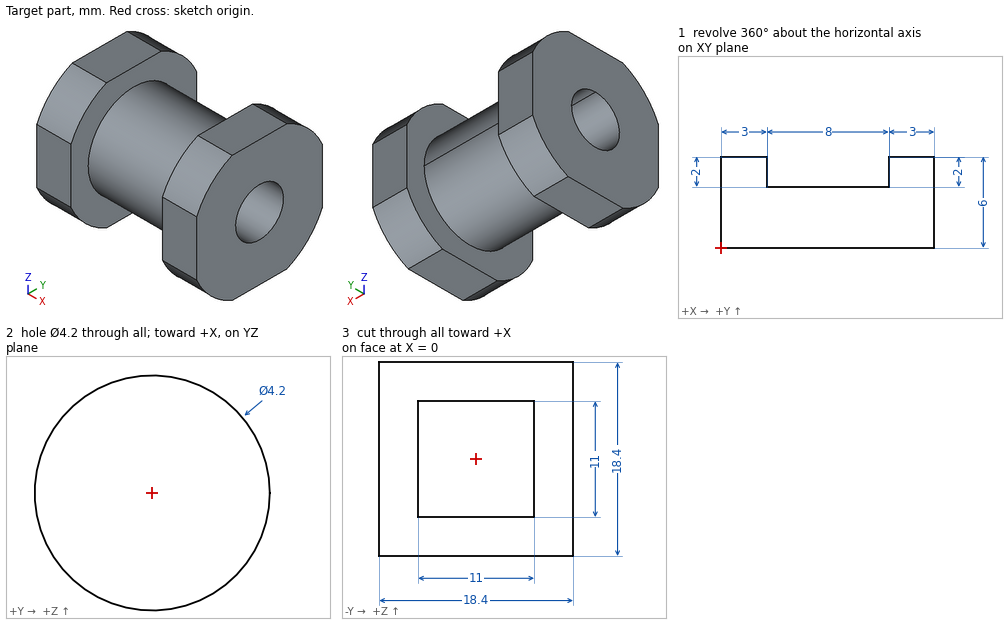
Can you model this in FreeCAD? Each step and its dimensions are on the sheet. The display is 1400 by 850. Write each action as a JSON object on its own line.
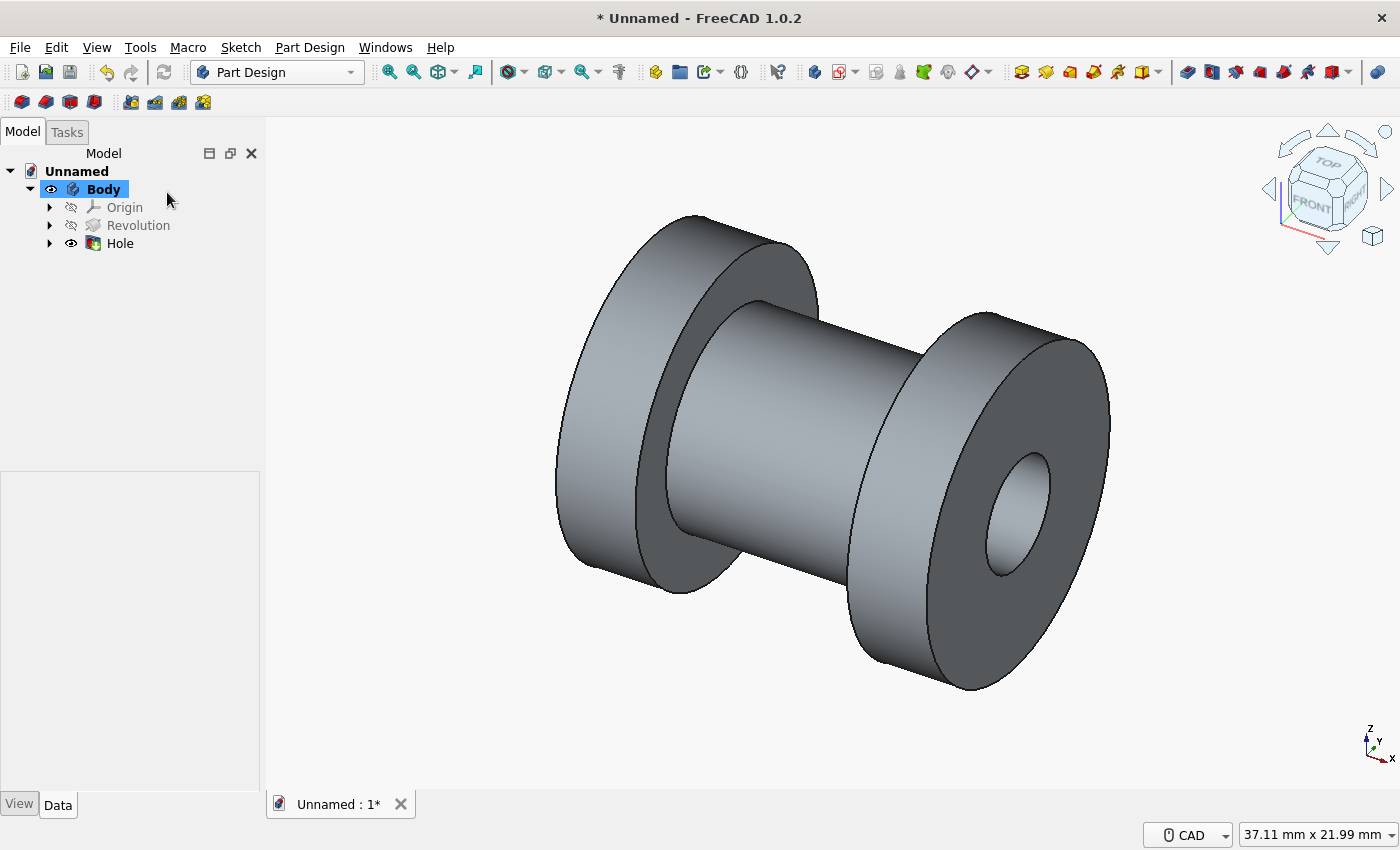
{"action": "key", "text": "6"}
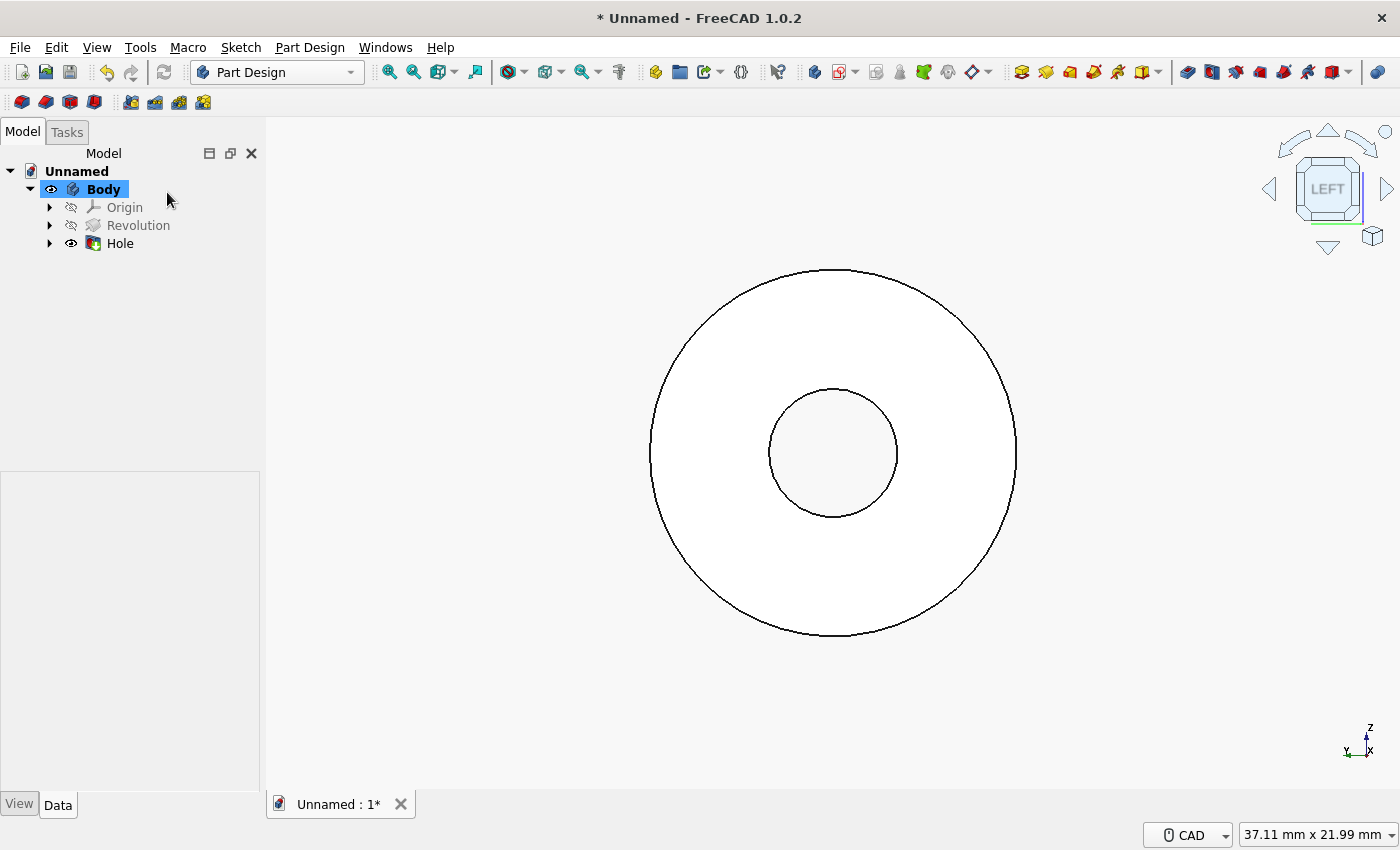
{"action": "left_click", "coordinate": [728, 504]}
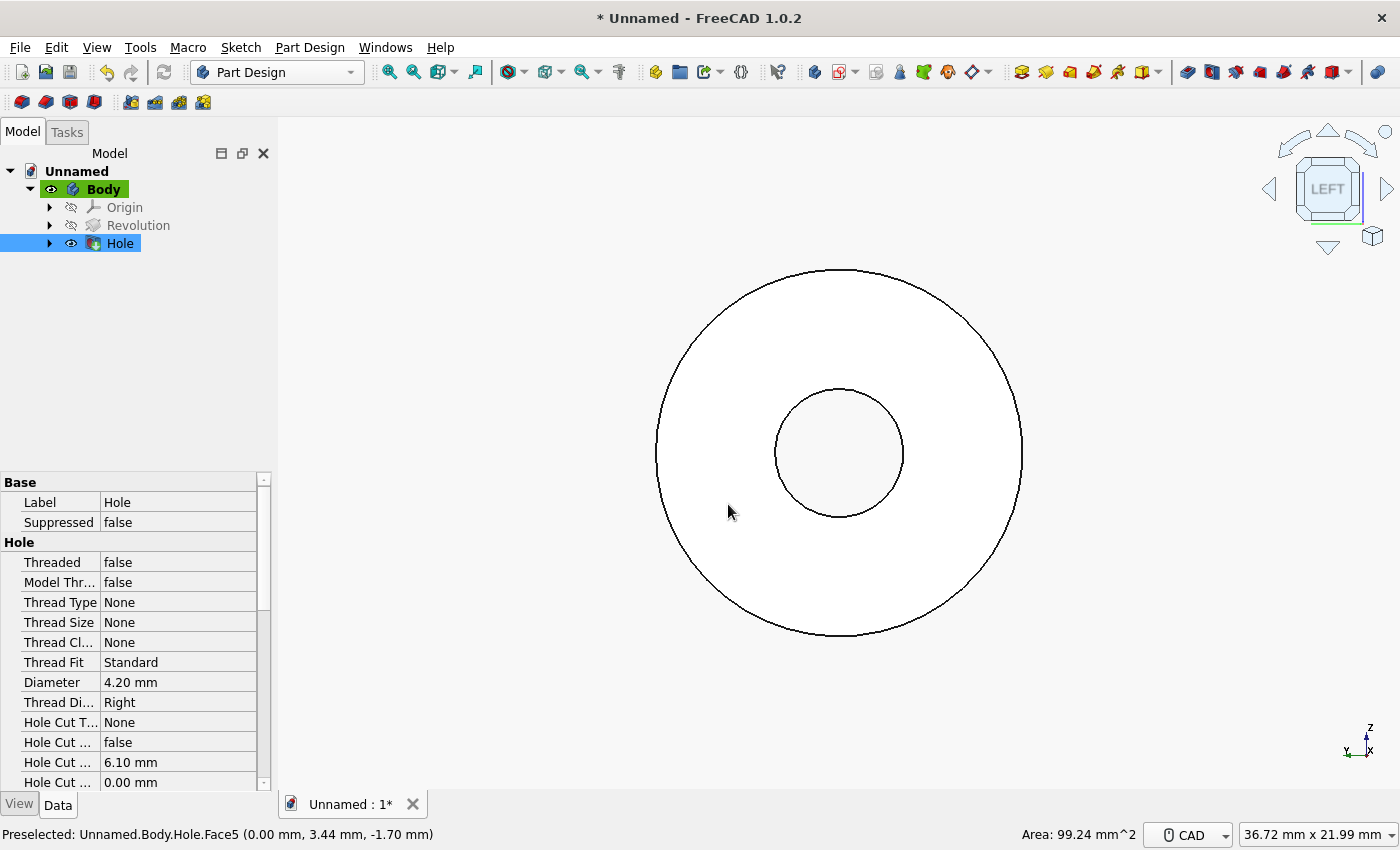
{"action": "left_click", "coordinate": [840, 72]}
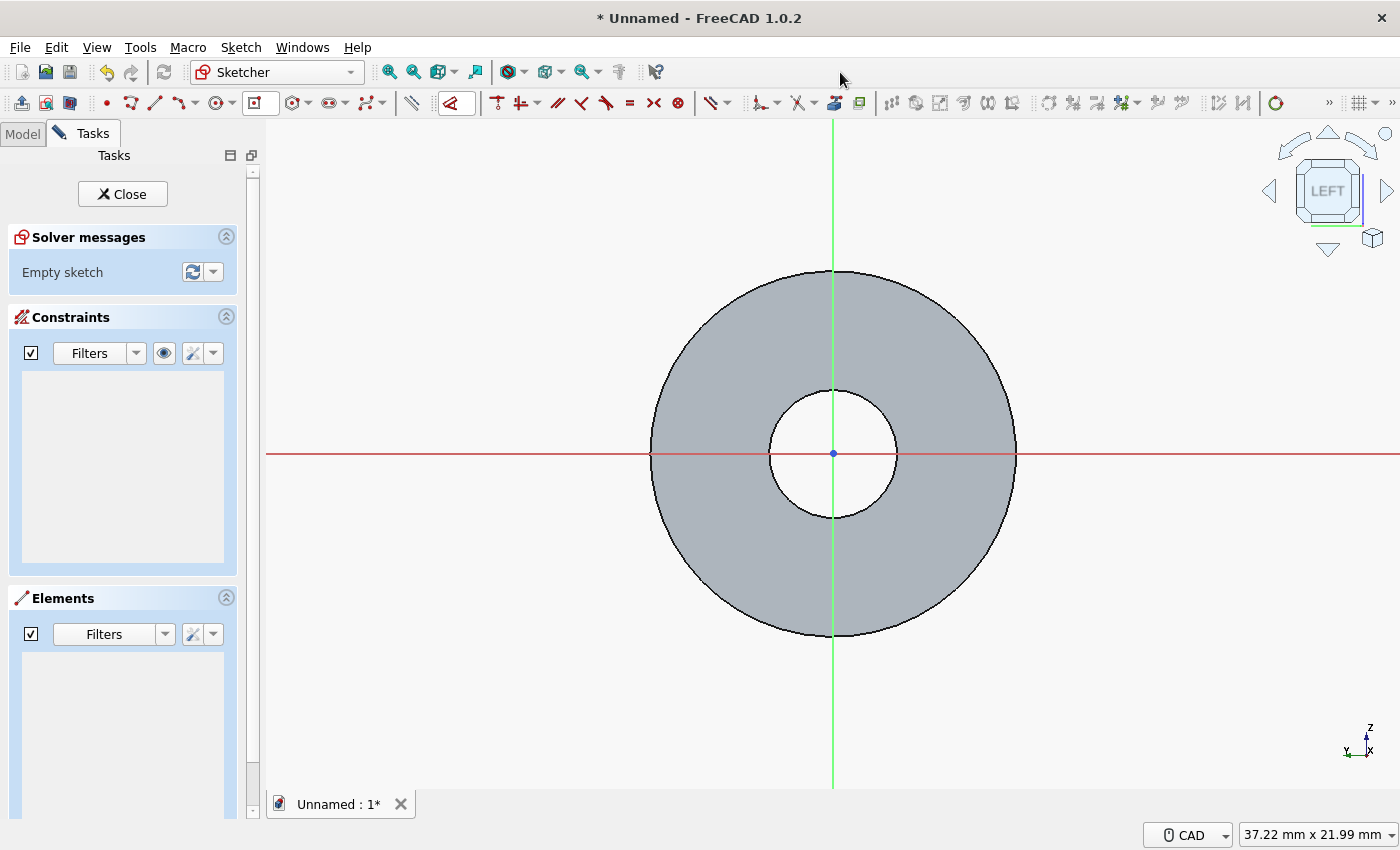
{"action": "left_click", "coordinate": [254, 104]}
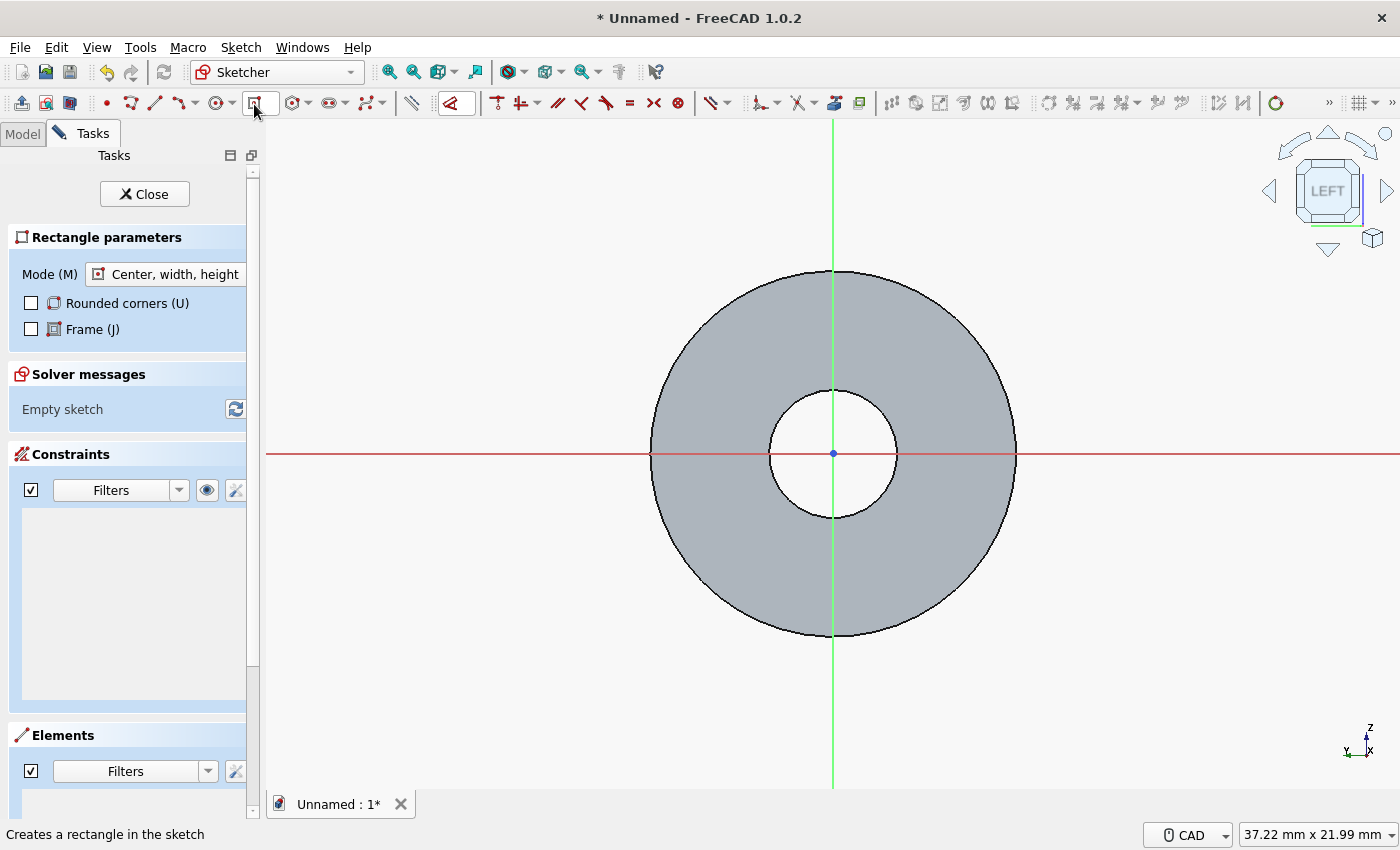
{"action": "left_click", "coordinate": [833, 454]}
{"action": "mouse_move", "coordinate": [1113, 174]}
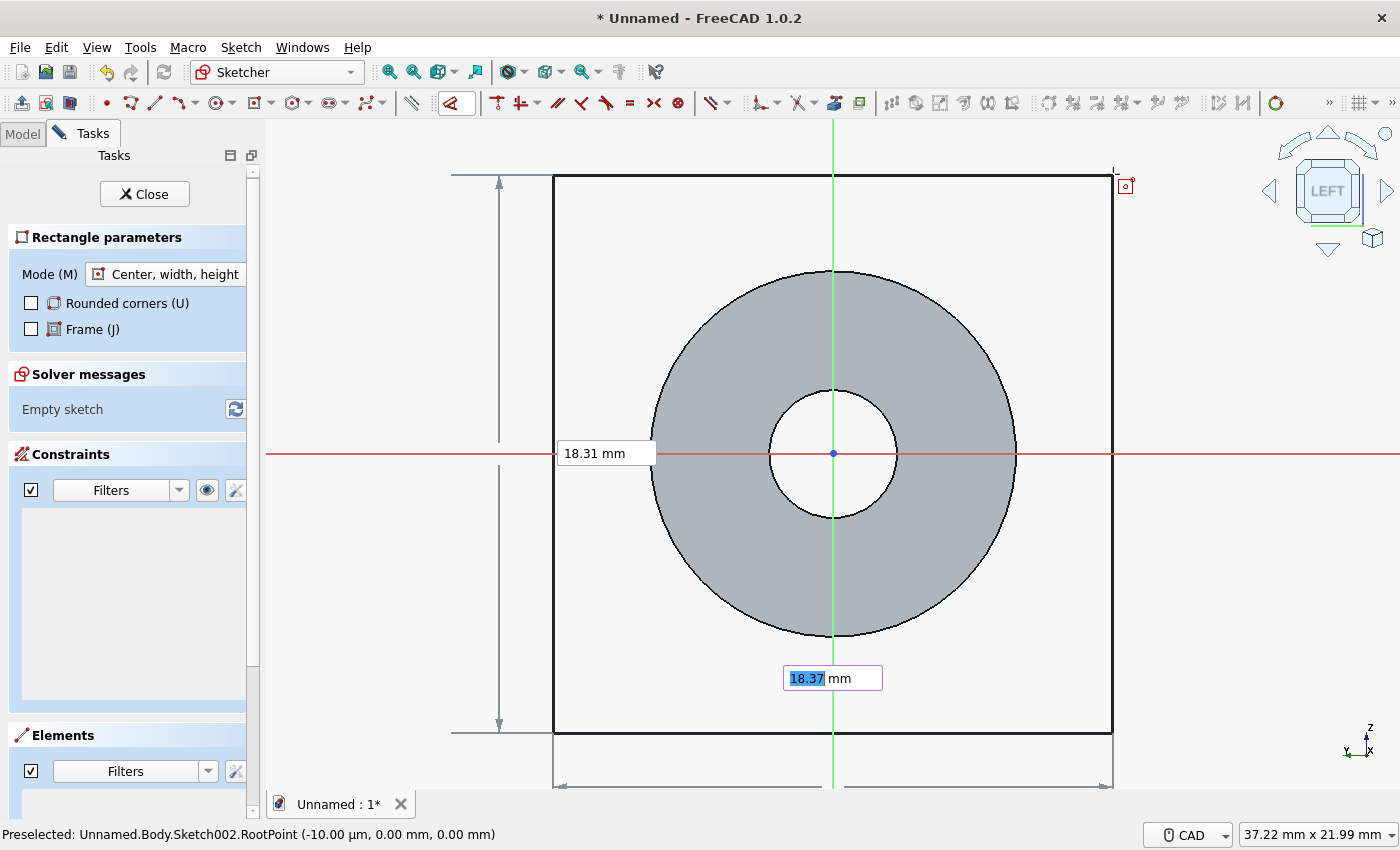
{"action": "type", "text": "18.4"}
{"action": "key", "text": "Tab"}
{"action": "type", "text": "18.4"}
{"action": "key", "text": "Return"}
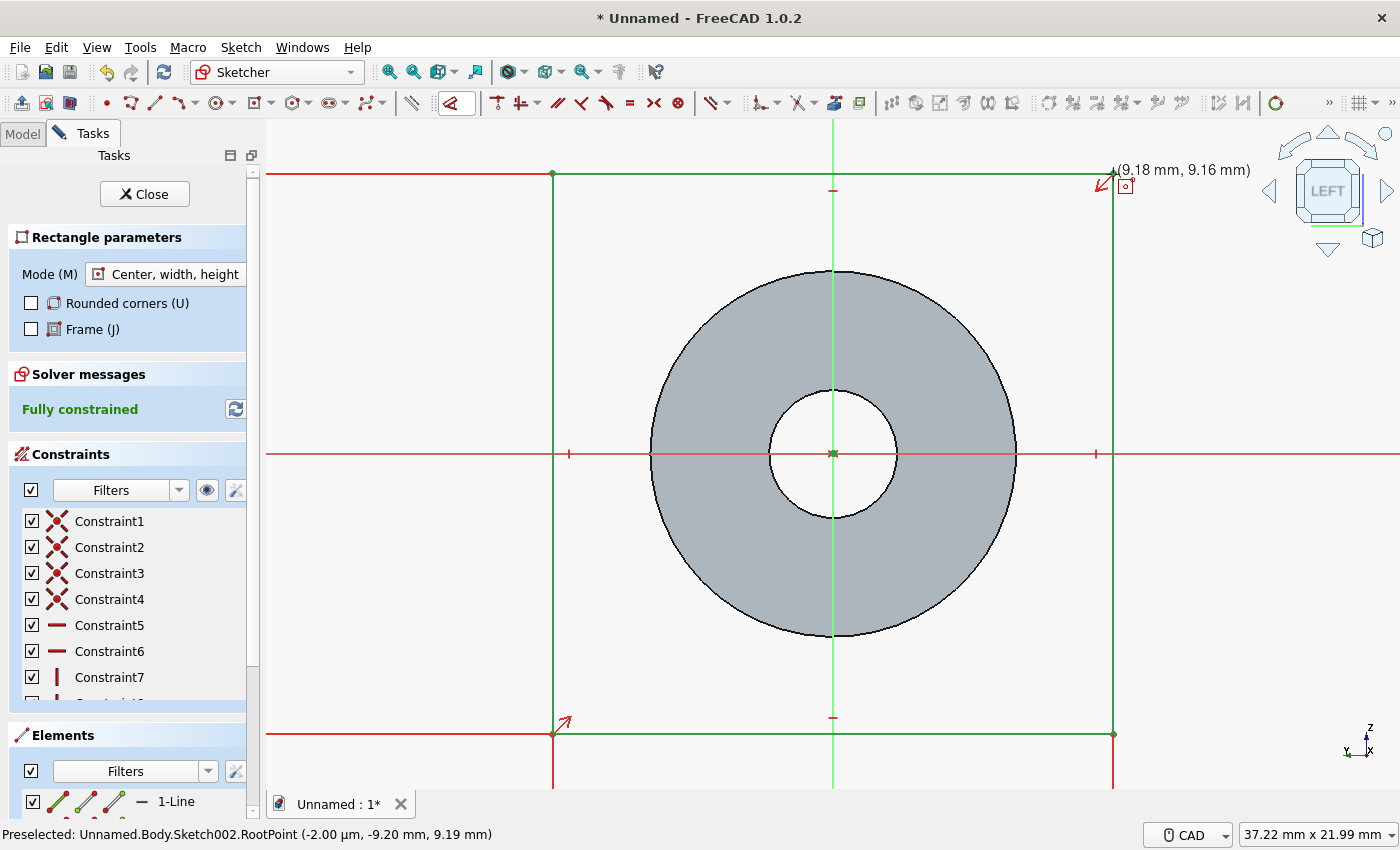
{"action": "left_click", "coordinate": [833, 454]}
{"action": "mouse_move", "coordinate": [1001, 286]}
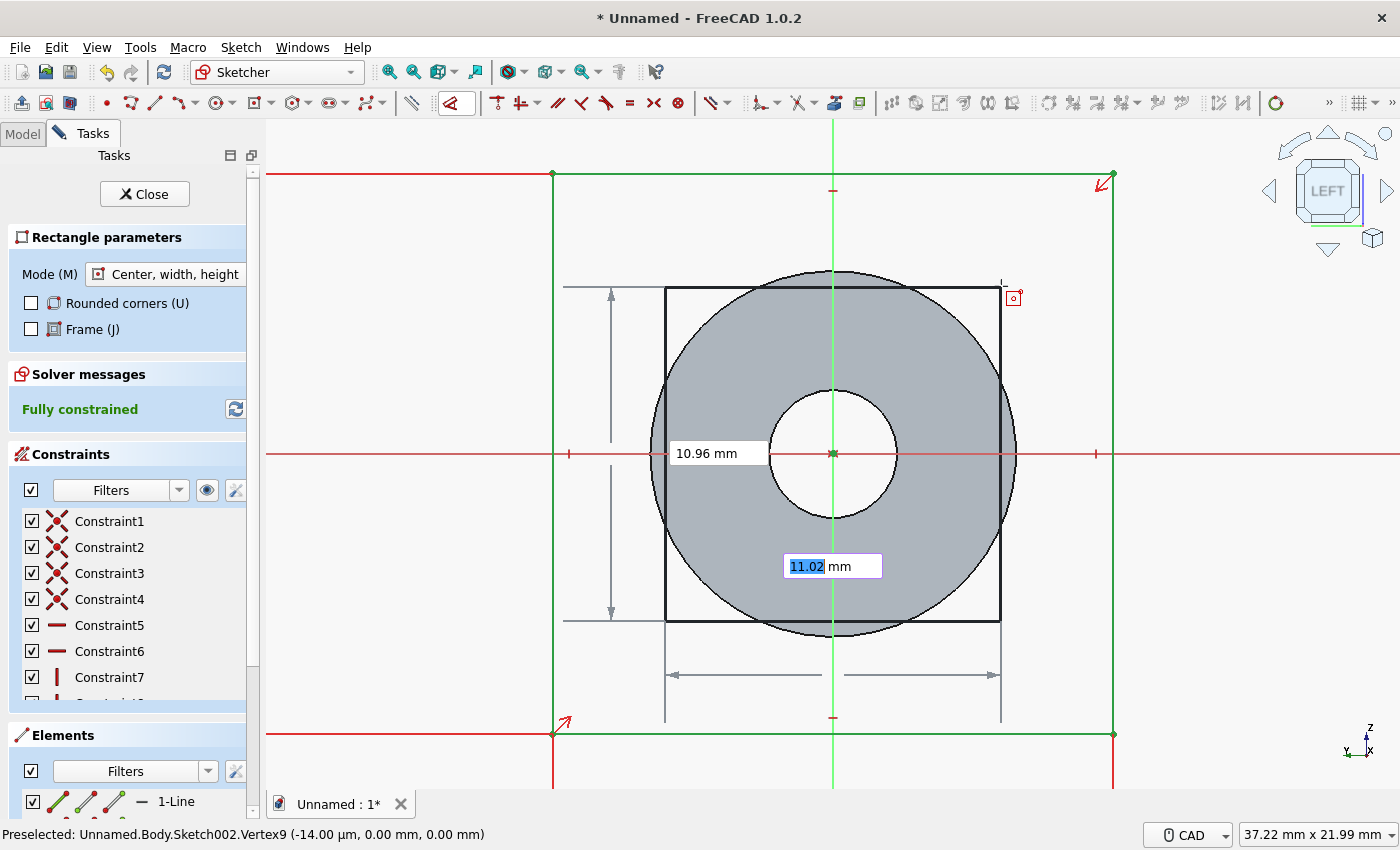
{"action": "type", "text": "11"}
{"action": "key", "text": "Tab"}
{"action": "type", "text": "11"}
{"action": "key", "text": "Return"}
{"action": "key", "text": "Escape"}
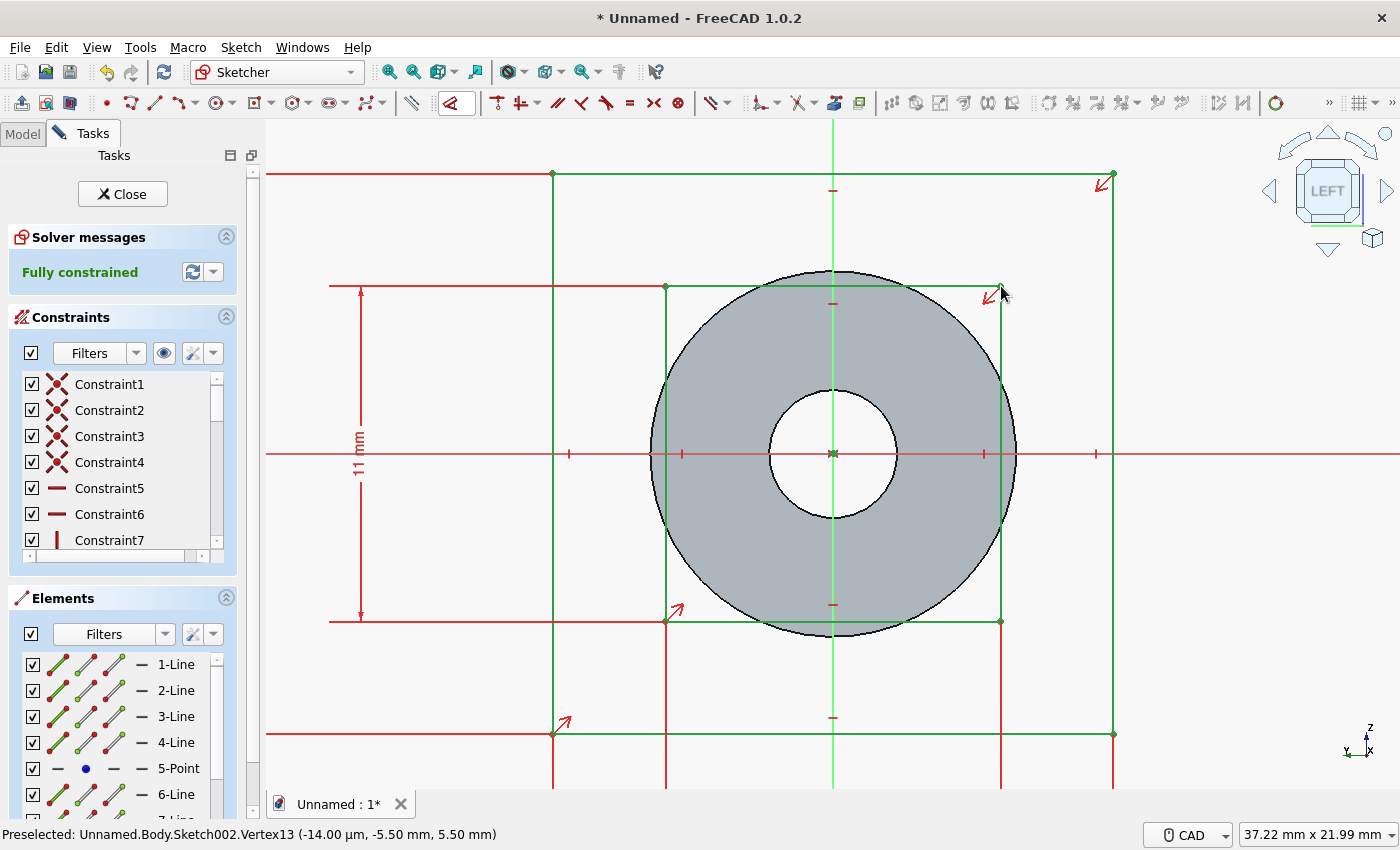
{"action": "left_click", "coordinate": [123, 194]}